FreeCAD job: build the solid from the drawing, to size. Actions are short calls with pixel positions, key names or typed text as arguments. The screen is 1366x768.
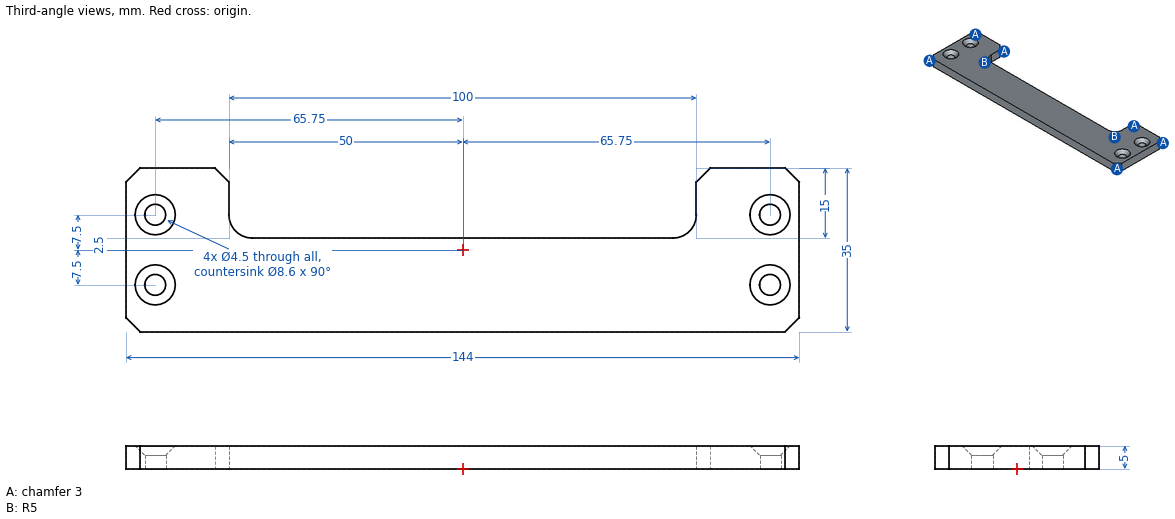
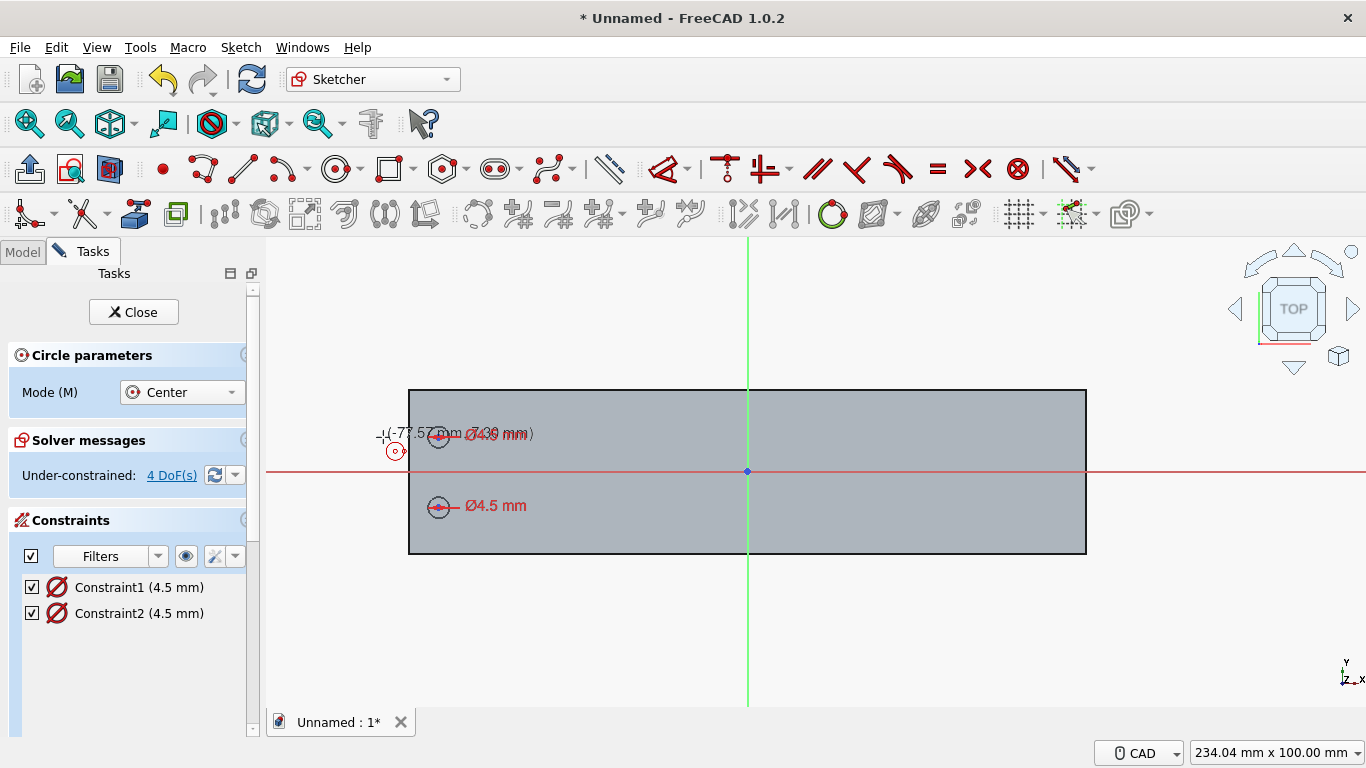
scroll(1057, 437, up, 4)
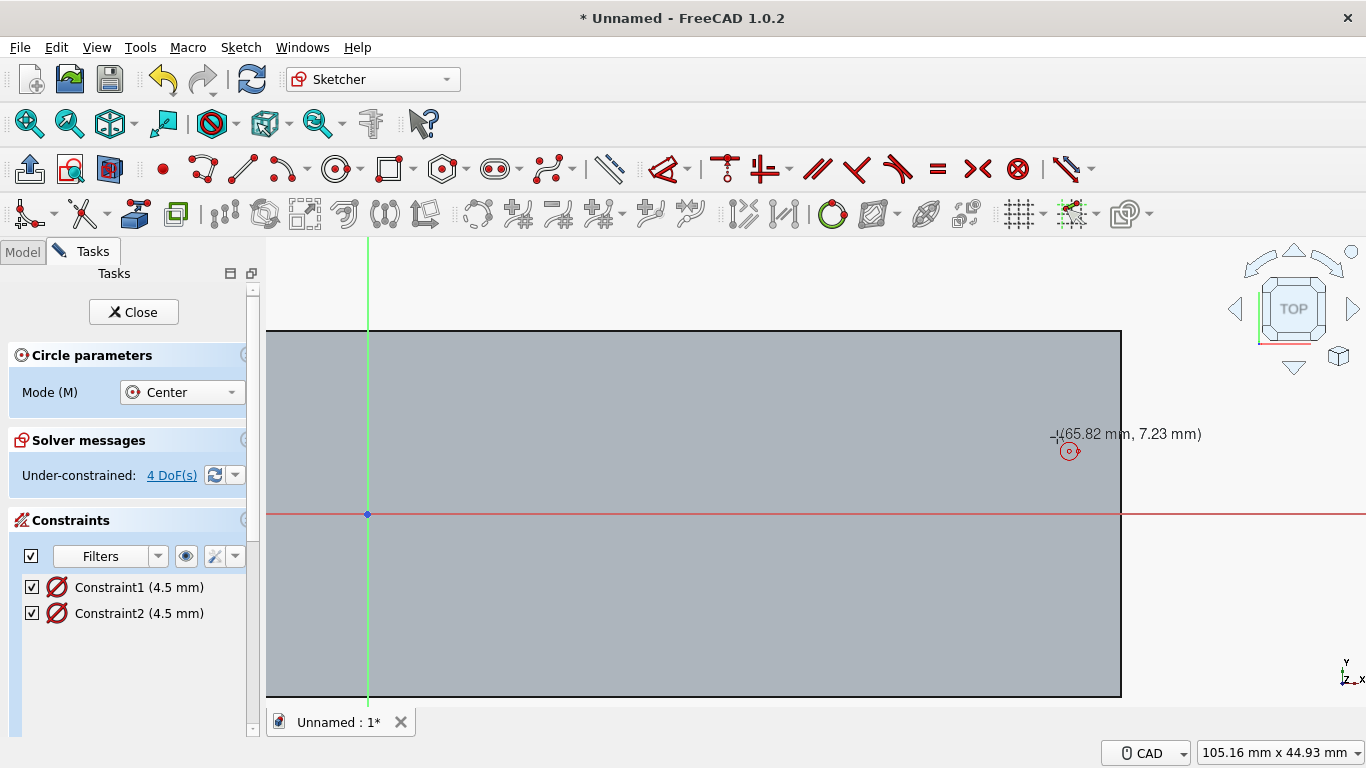
click(1055, 436)
move(1072, 419)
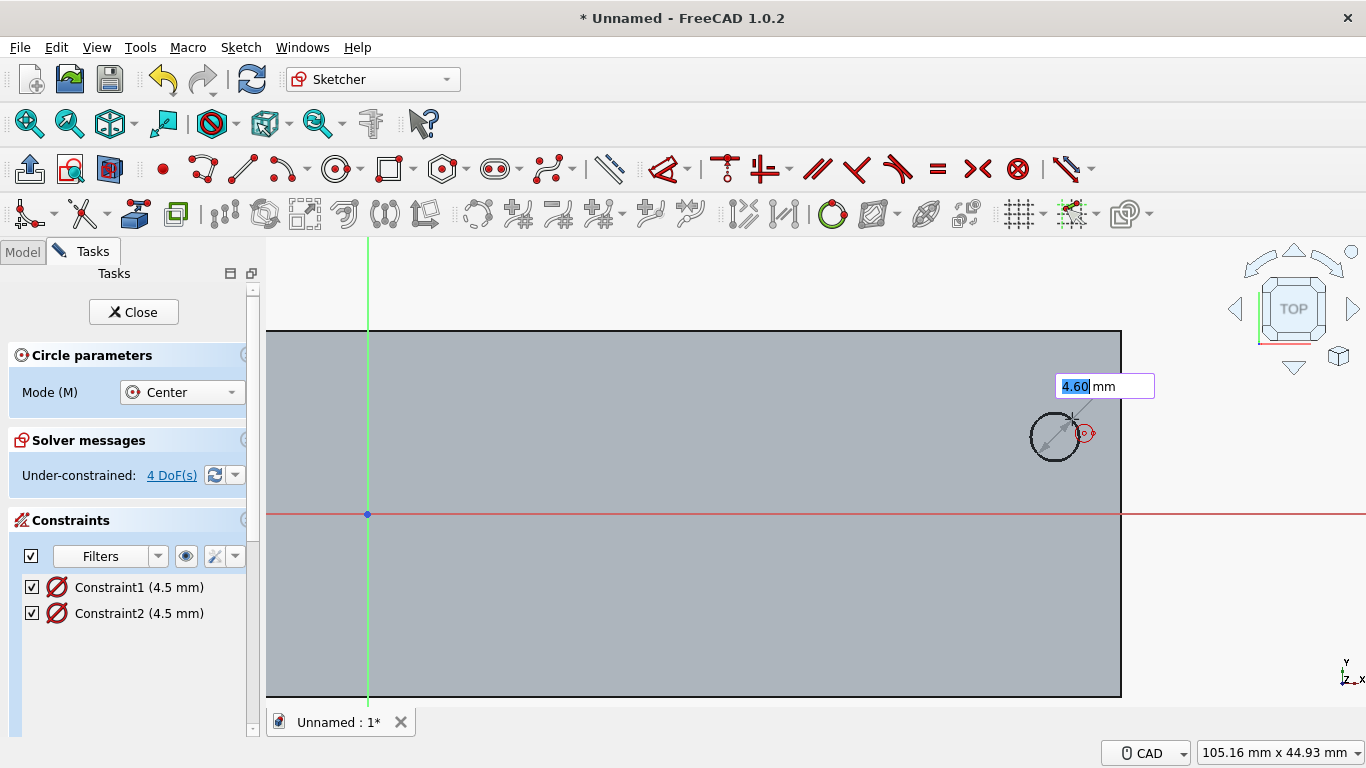
text(4.5)
key(Return)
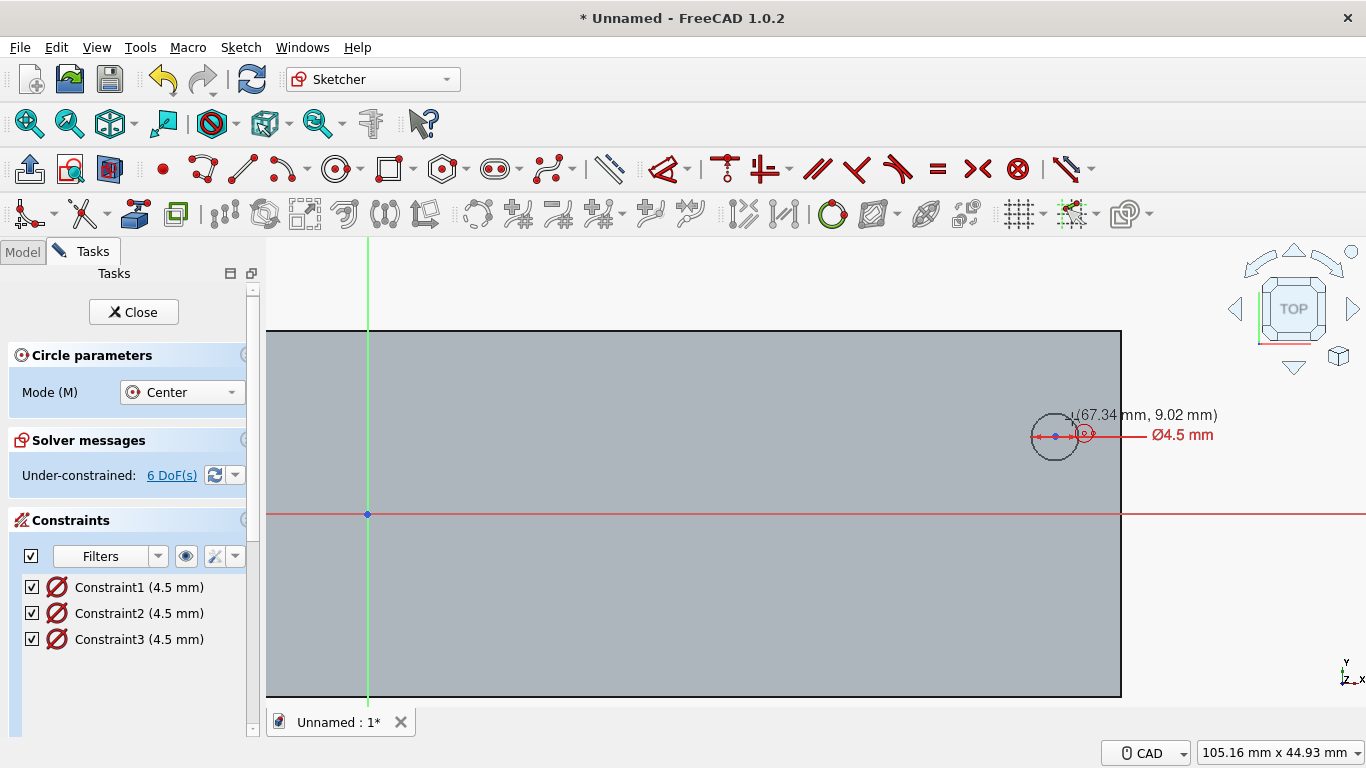
click(1055, 593)
move(1072, 576)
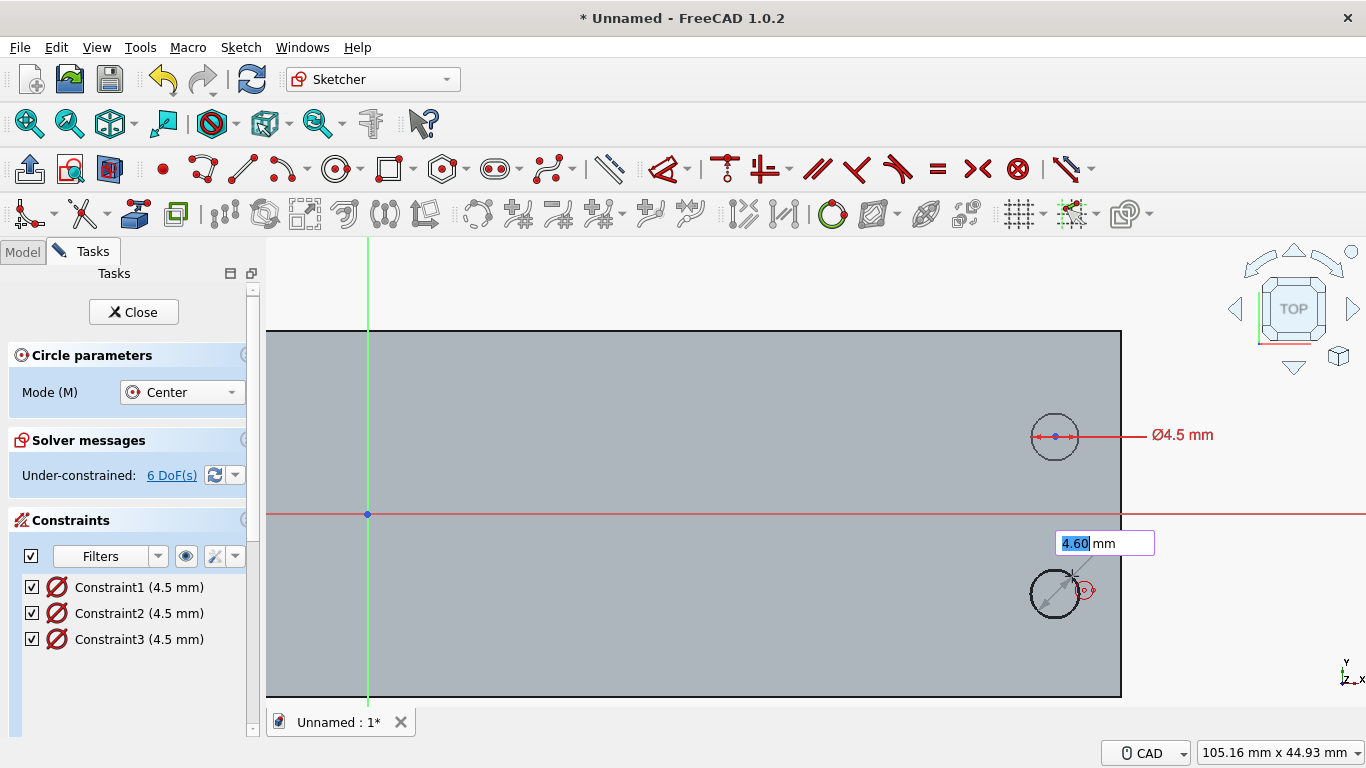
text(4.5)
key(Return)
key(Escape)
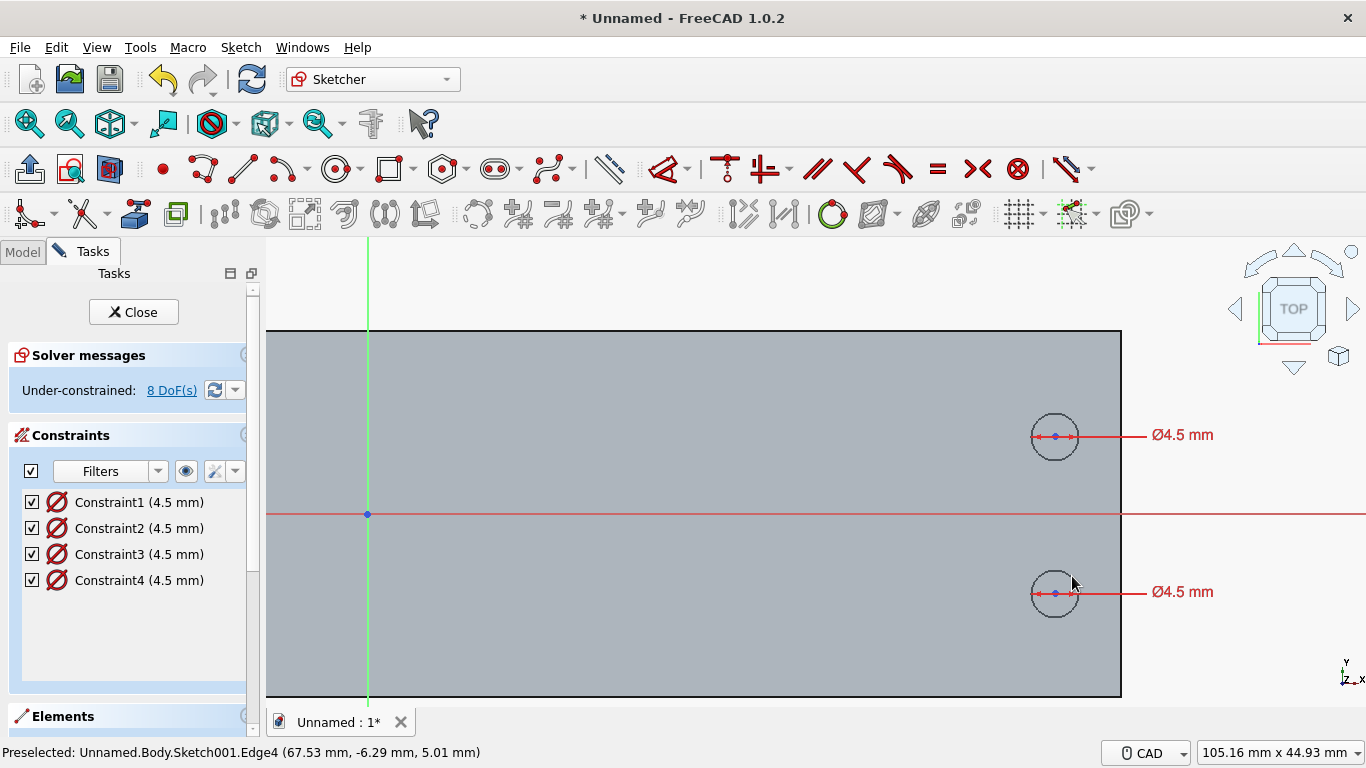
key(d)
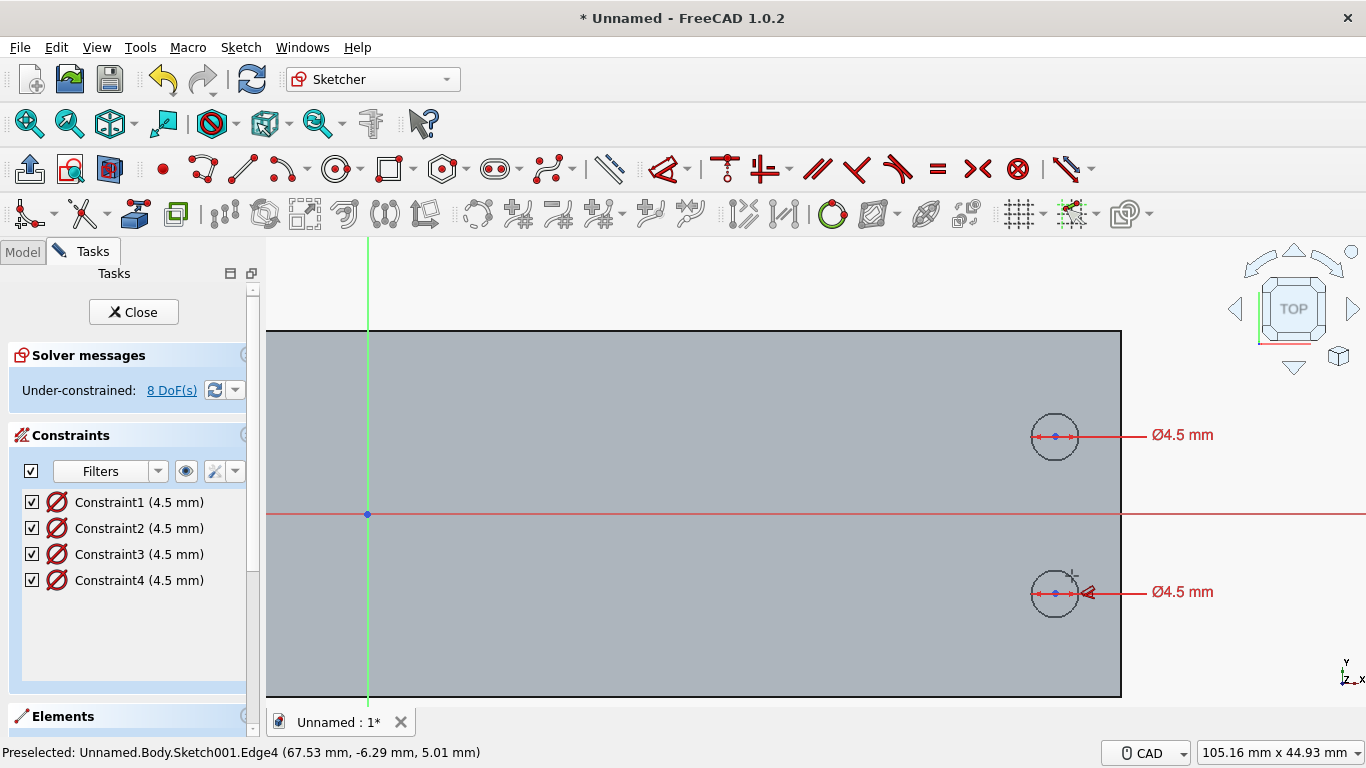
scroll(1057, 437, down, 4)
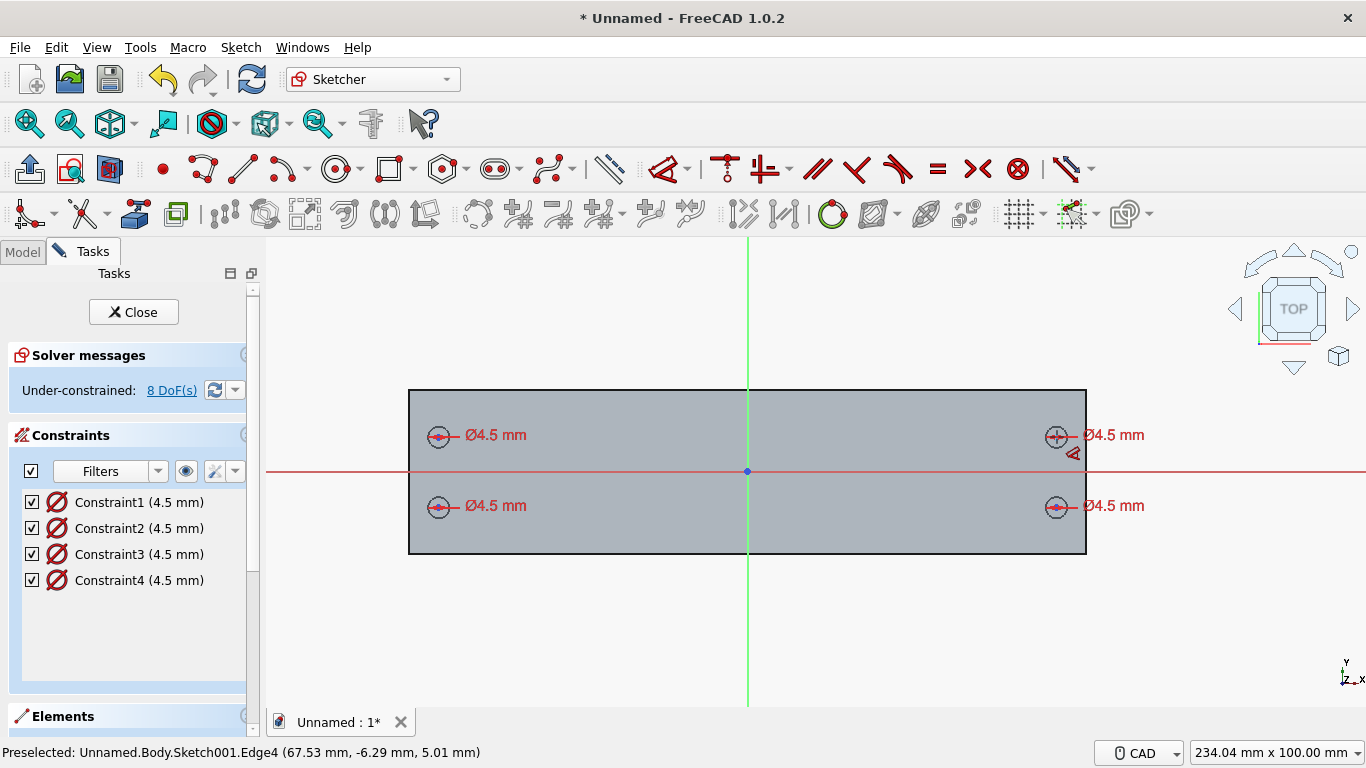
click(439, 437)
click(405, 455)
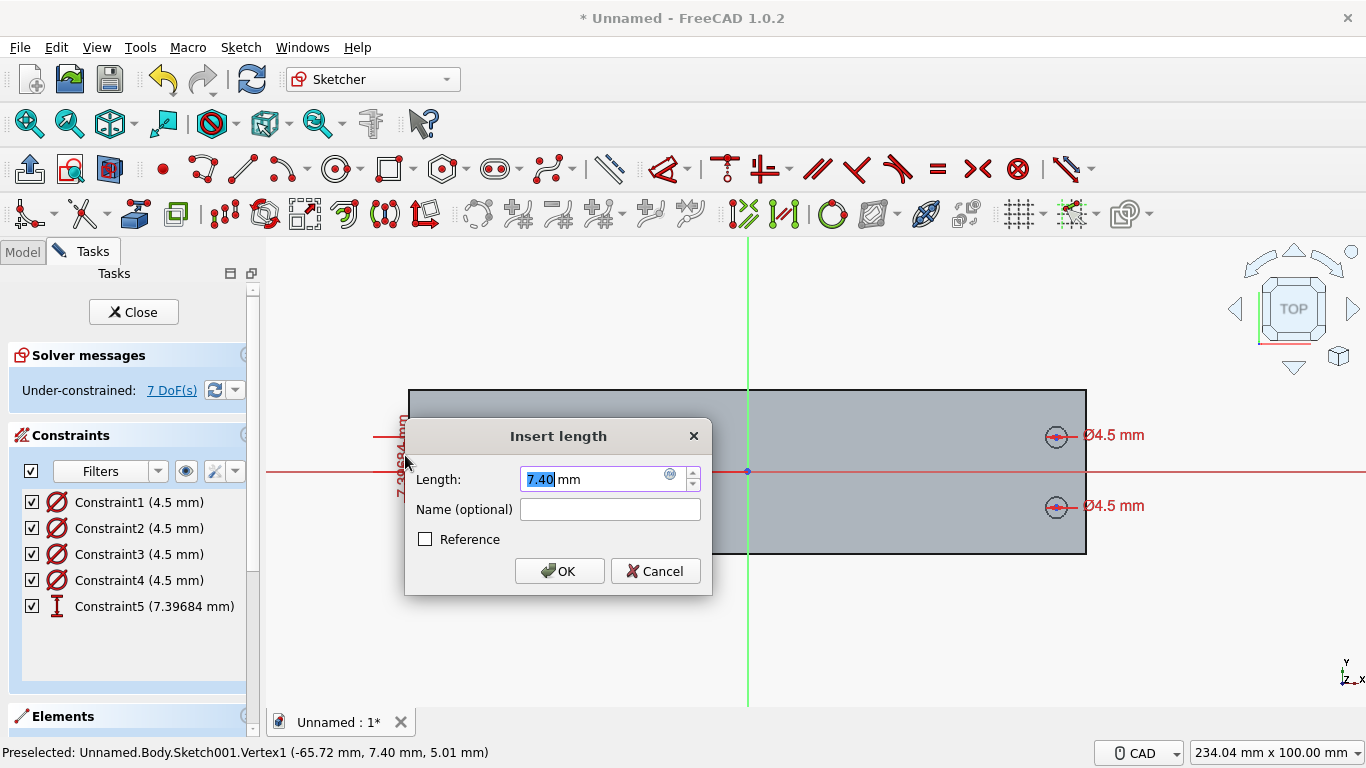
text(7.5)
key(Return)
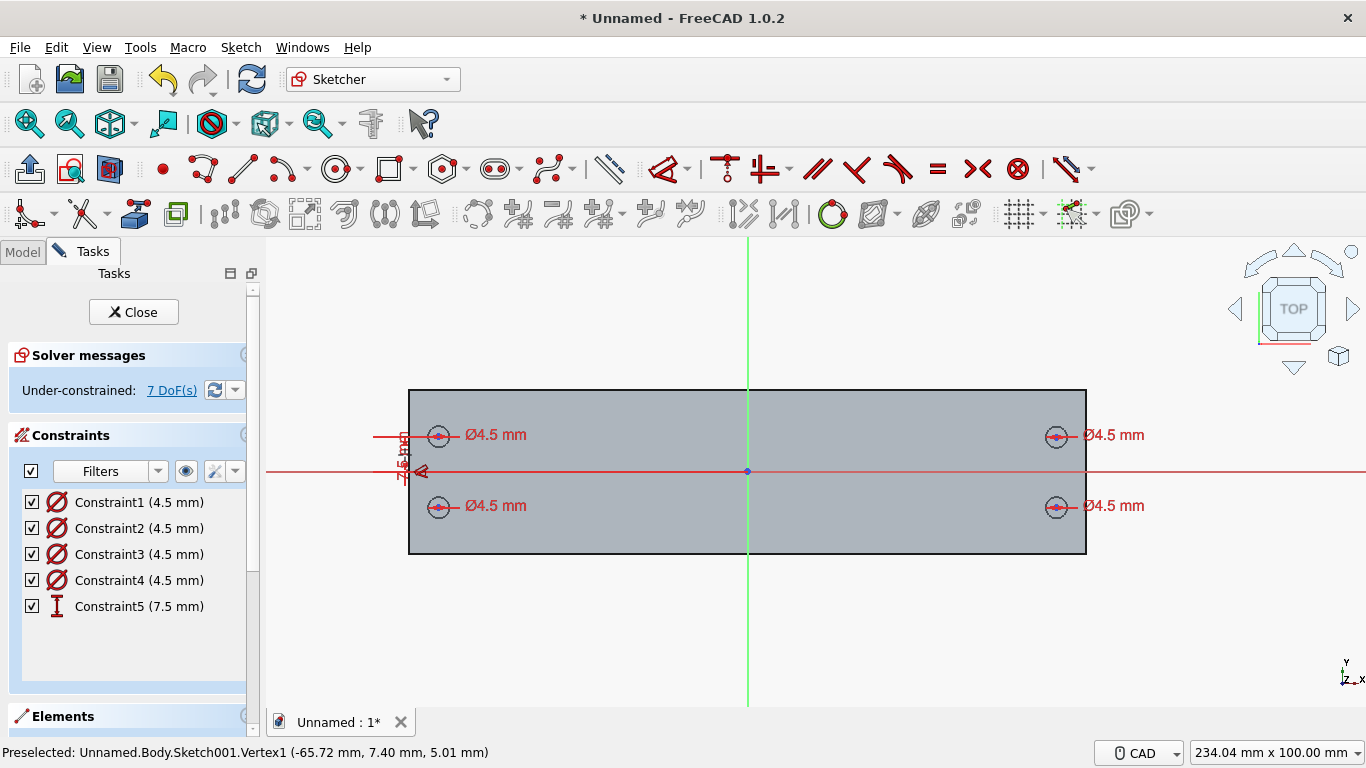
click(439, 508)
click(405, 490)